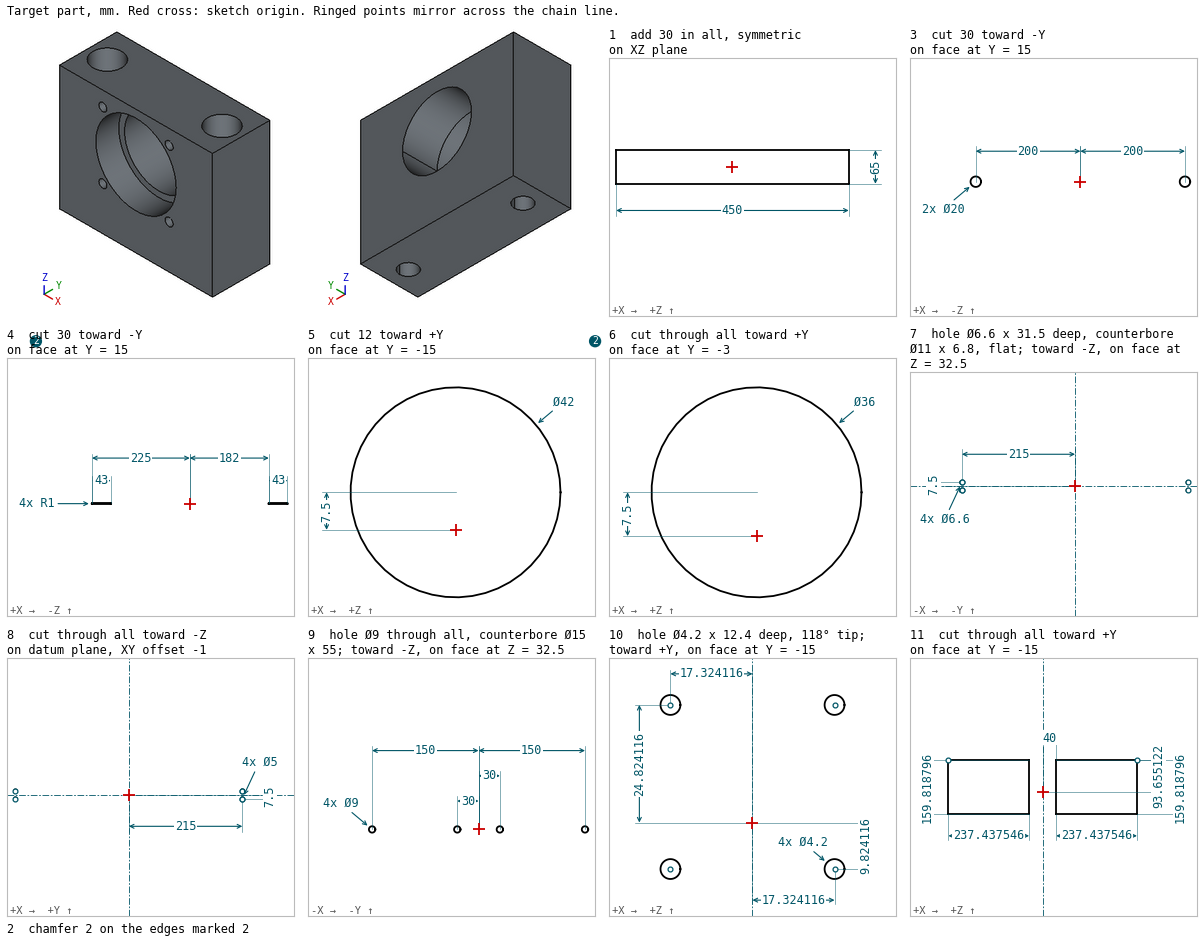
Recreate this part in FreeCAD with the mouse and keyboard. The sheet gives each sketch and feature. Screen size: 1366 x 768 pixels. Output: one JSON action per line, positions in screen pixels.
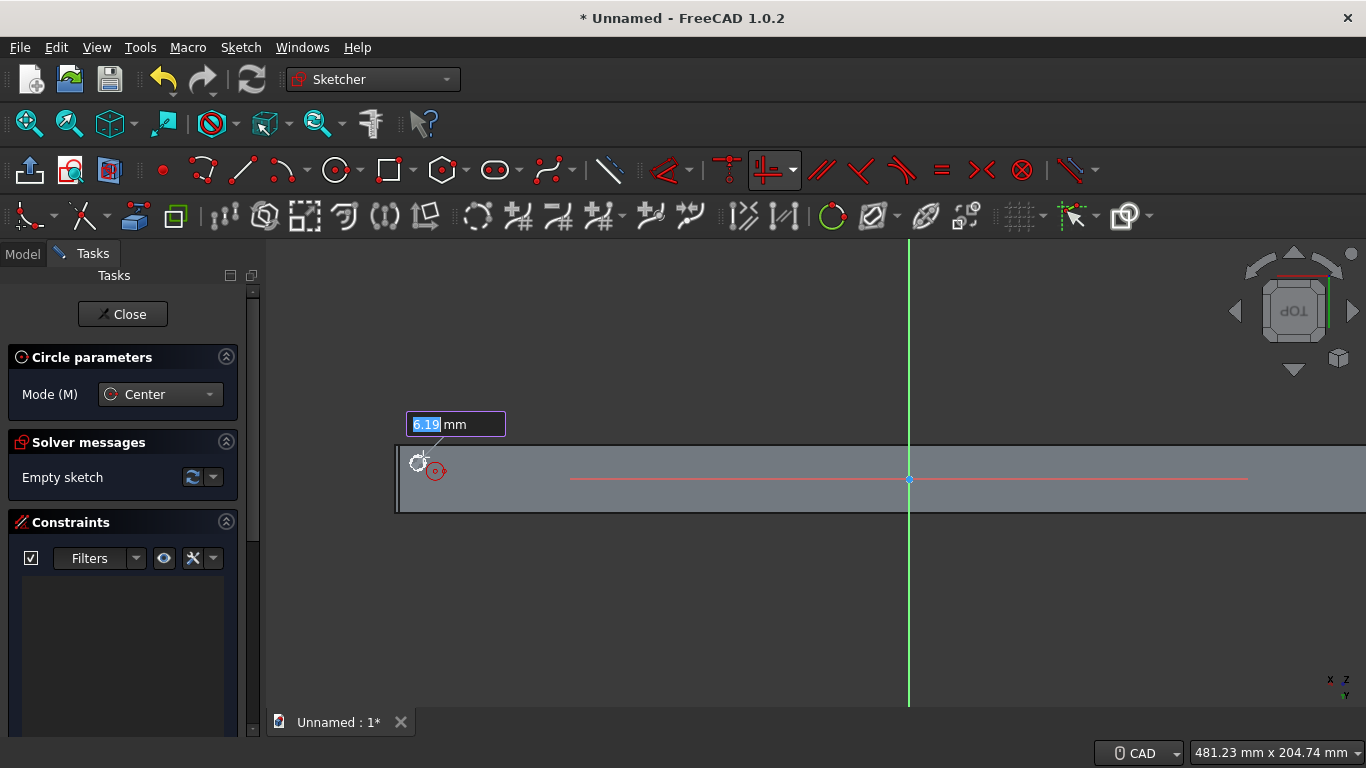
{"action": "type", "text": "6.6"}
{"action": "key", "text": "Return"}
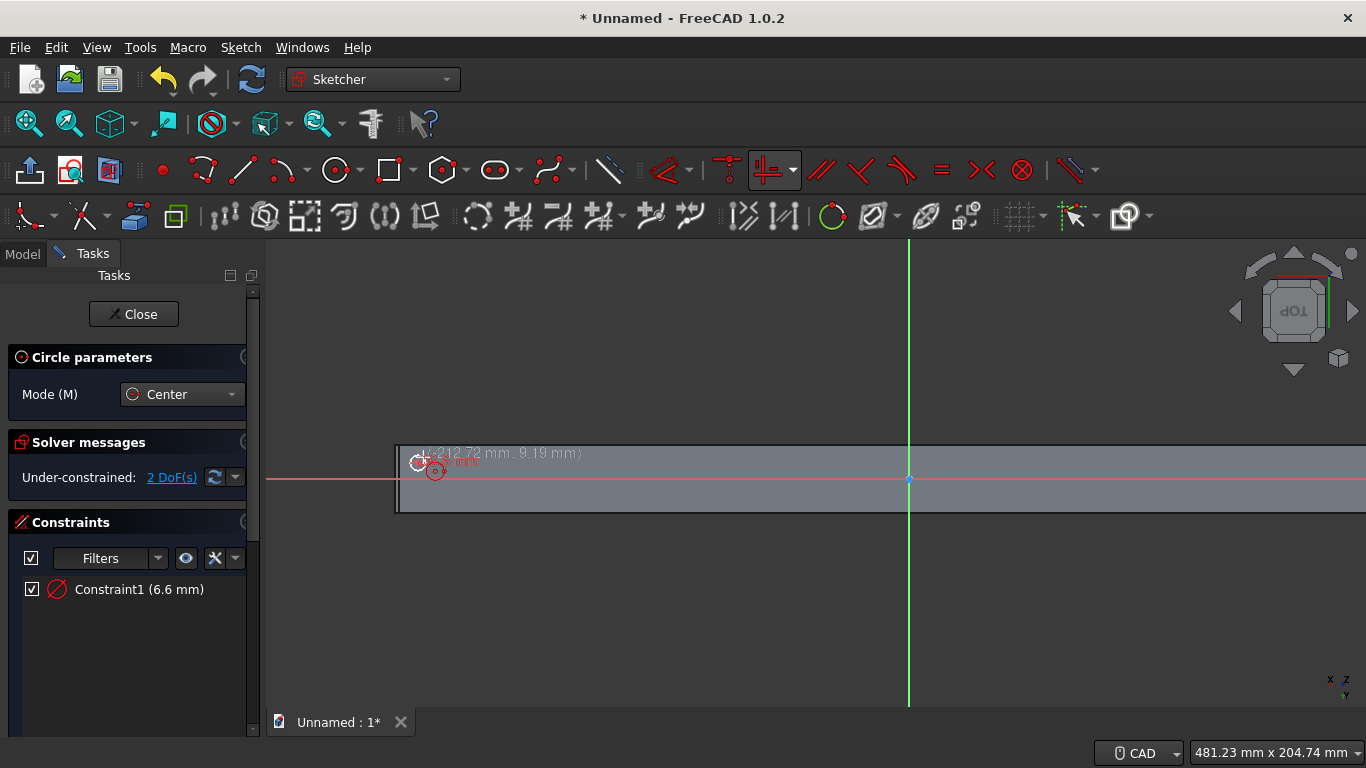
{"action": "scroll", "coordinate": [418, 496], "scroll_direction": "up", "scroll_amount": 6}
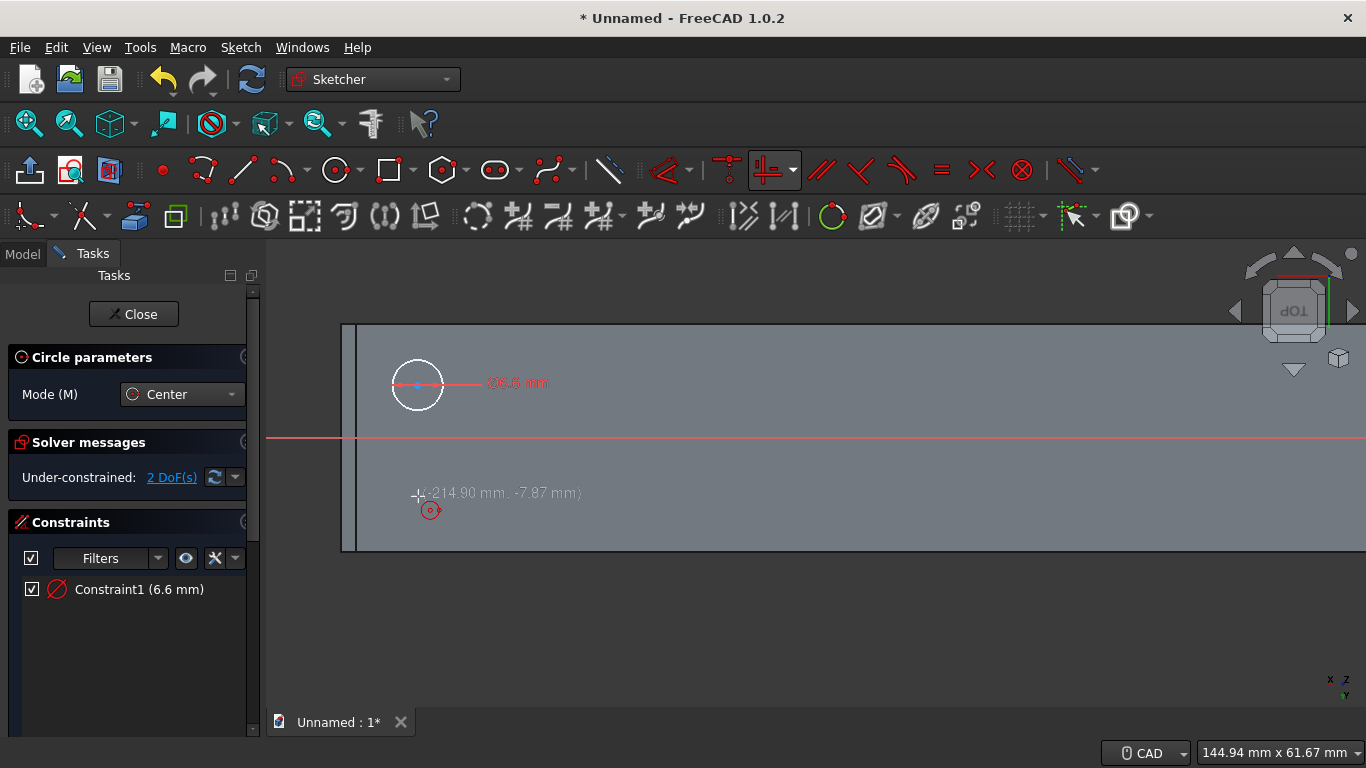
{"action": "scroll", "coordinate": [418, 482], "scroll_direction": "down", "scroll_amount": 8}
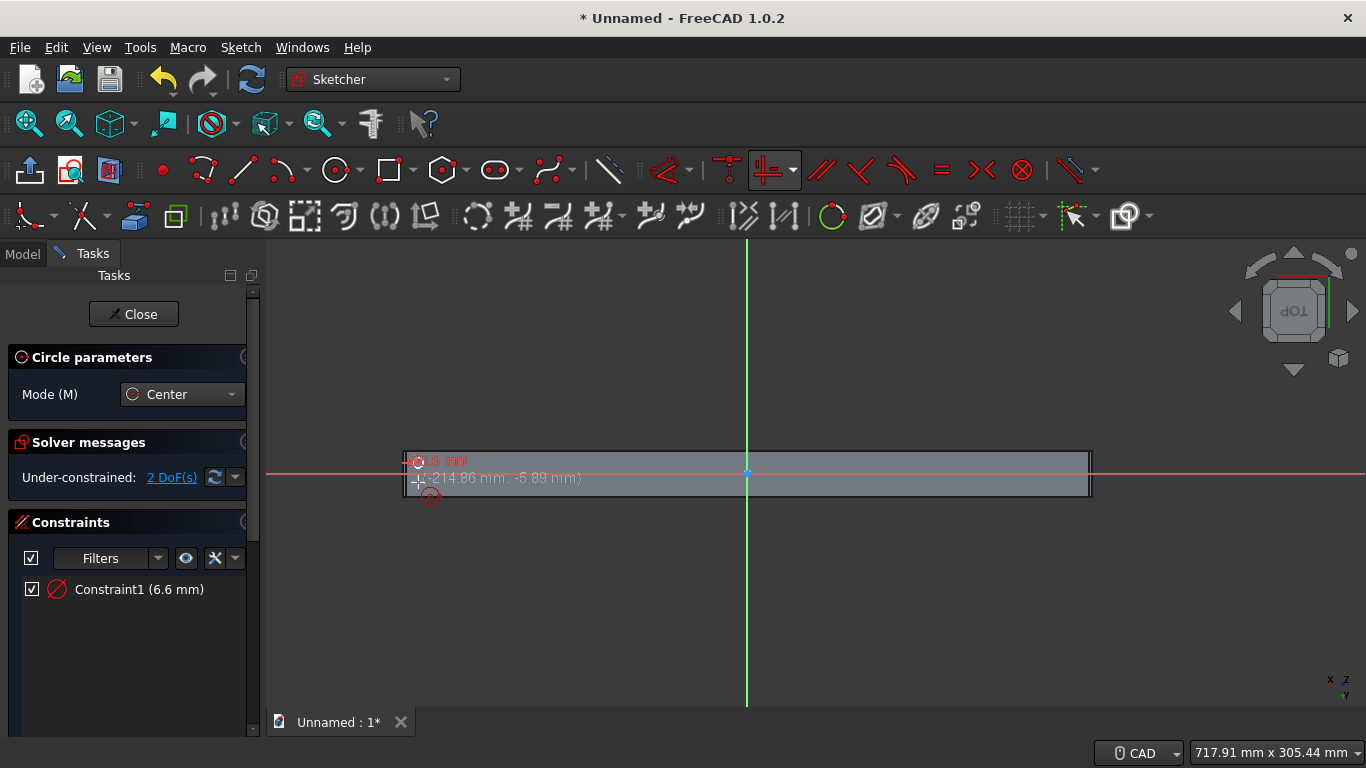
{"action": "scroll", "coordinate": [418, 485], "scroll_direction": "up", "scroll_amount": 2}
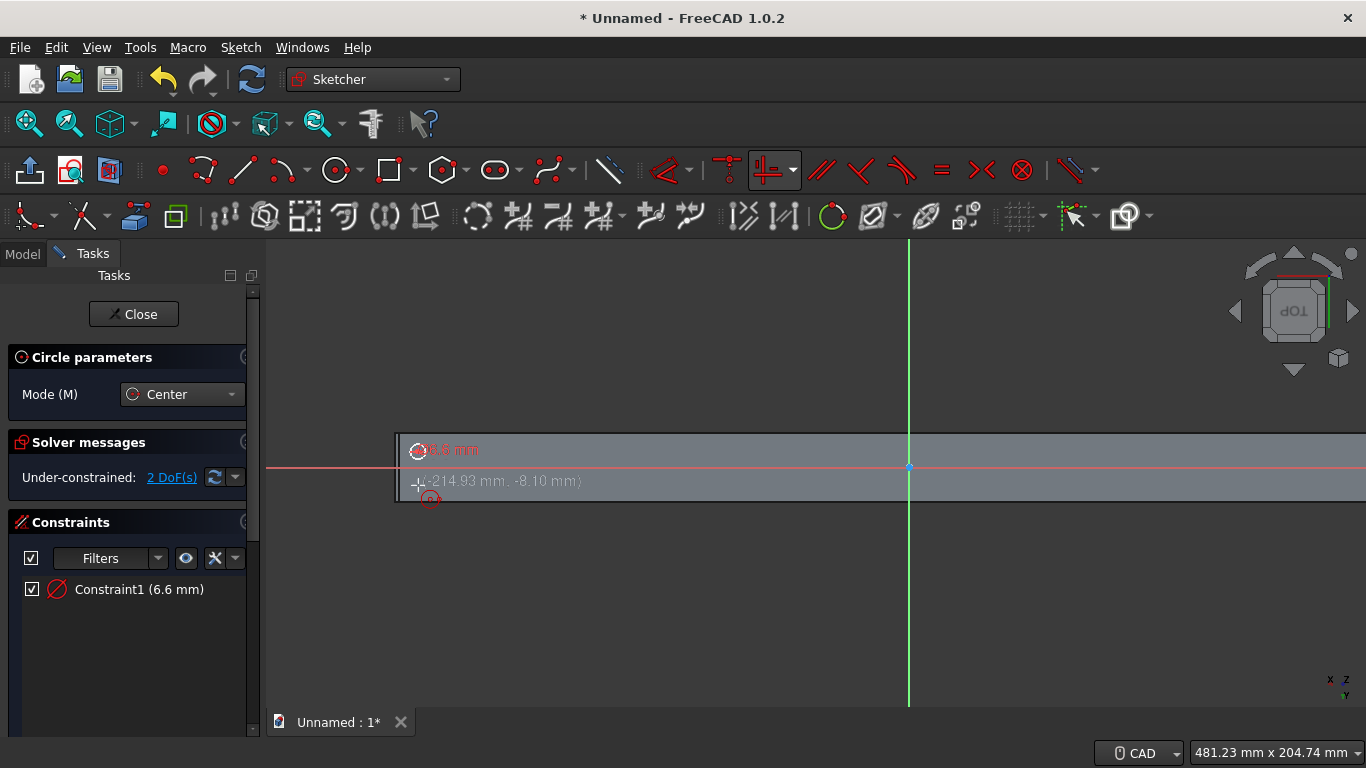
{"action": "left_click", "coordinate": [418, 485]}
{"action": "mouse_move", "coordinate": [423, 490]}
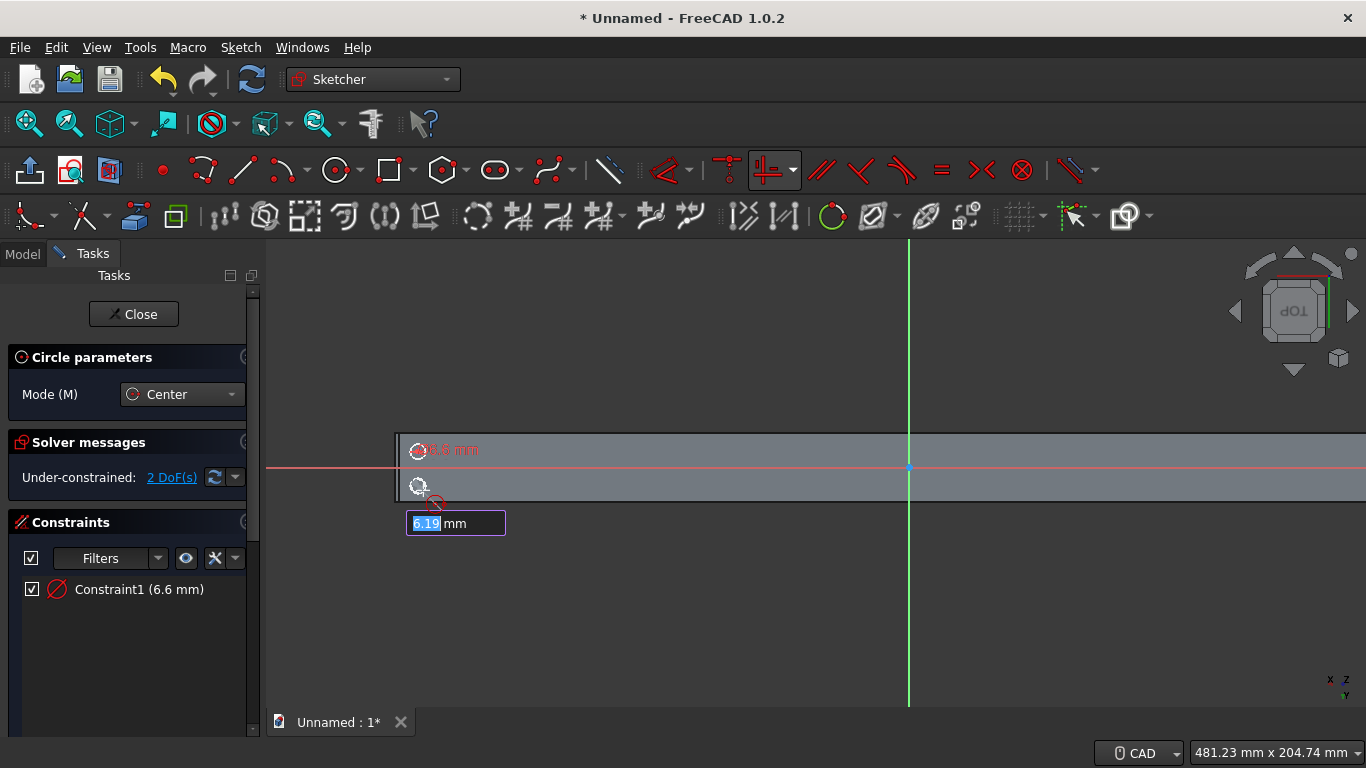
{"action": "type", "text": "6.6"}
{"action": "key", "text": "Return"}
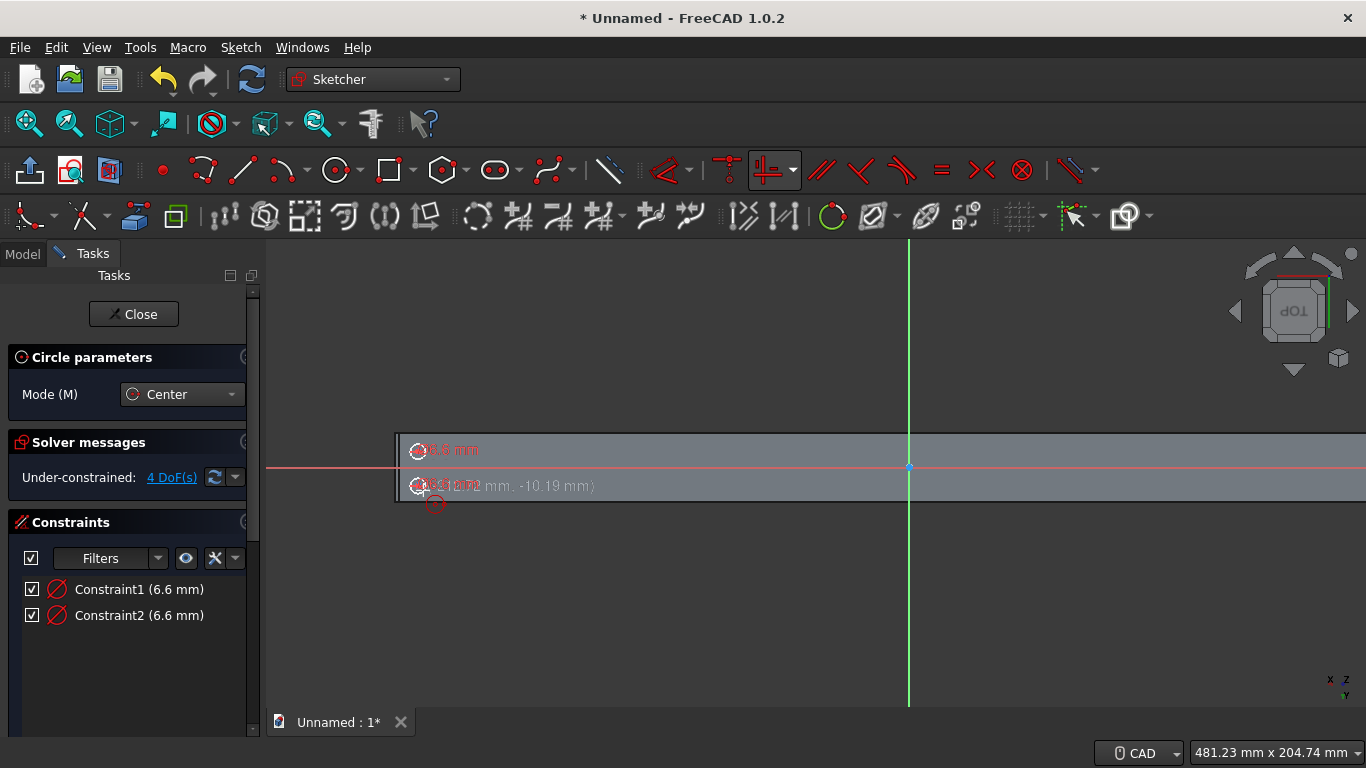
{"action": "scroll", "coordinate": [419, 484], "scroll_direction": "down", "scroll_amount": 2}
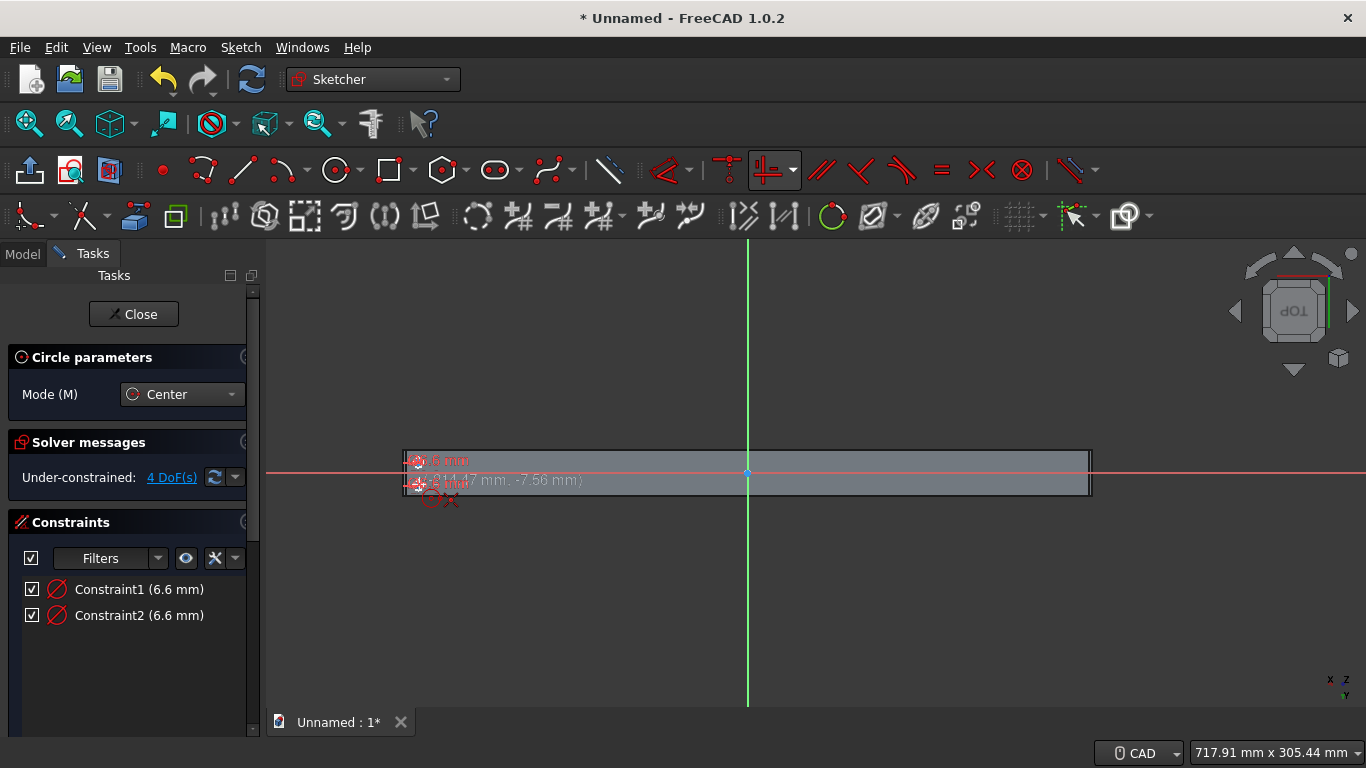
{"action": "scroll", "coordinate": [1077, 485], "scroll_direction": "up", "scroll_amount": 8}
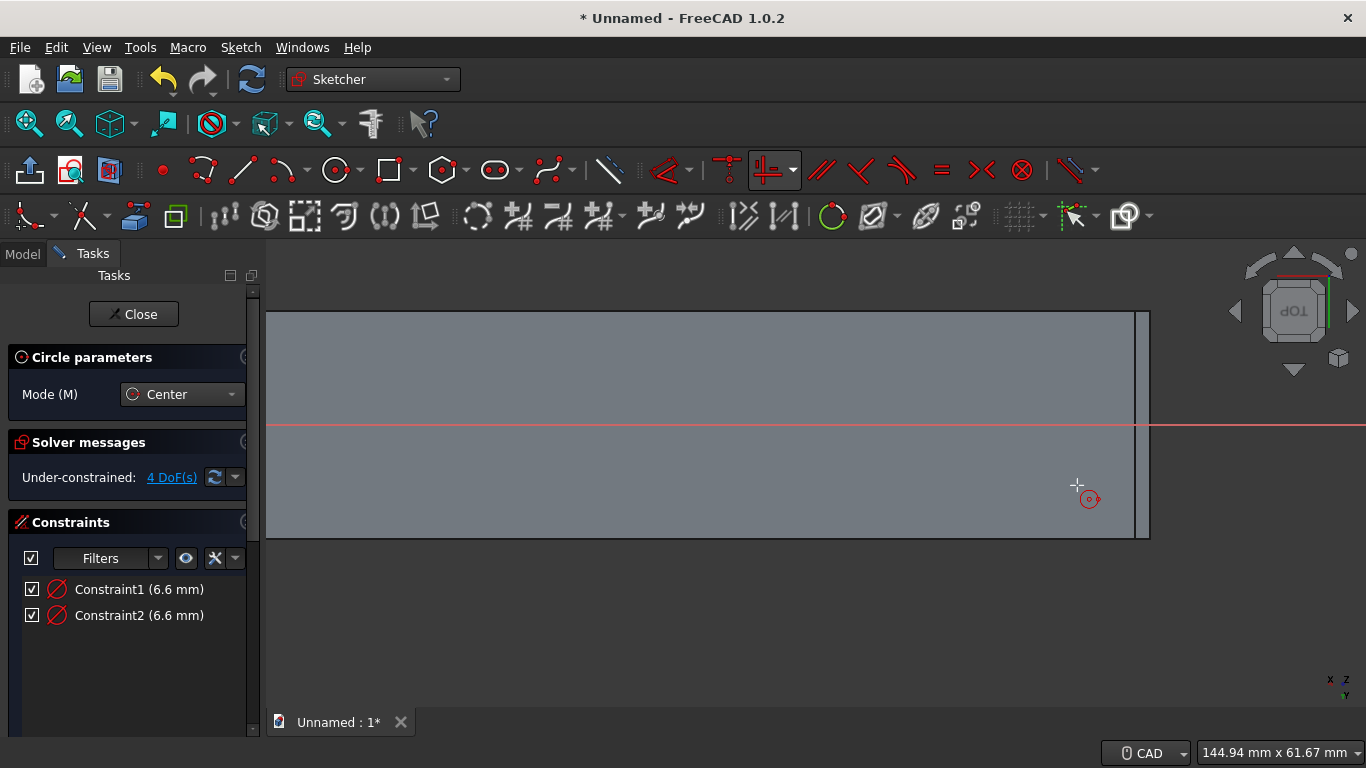
{"action": "scroll", "coordinate": [1078, 485], "scroll_direction": "down", "scroll_amount": 8}